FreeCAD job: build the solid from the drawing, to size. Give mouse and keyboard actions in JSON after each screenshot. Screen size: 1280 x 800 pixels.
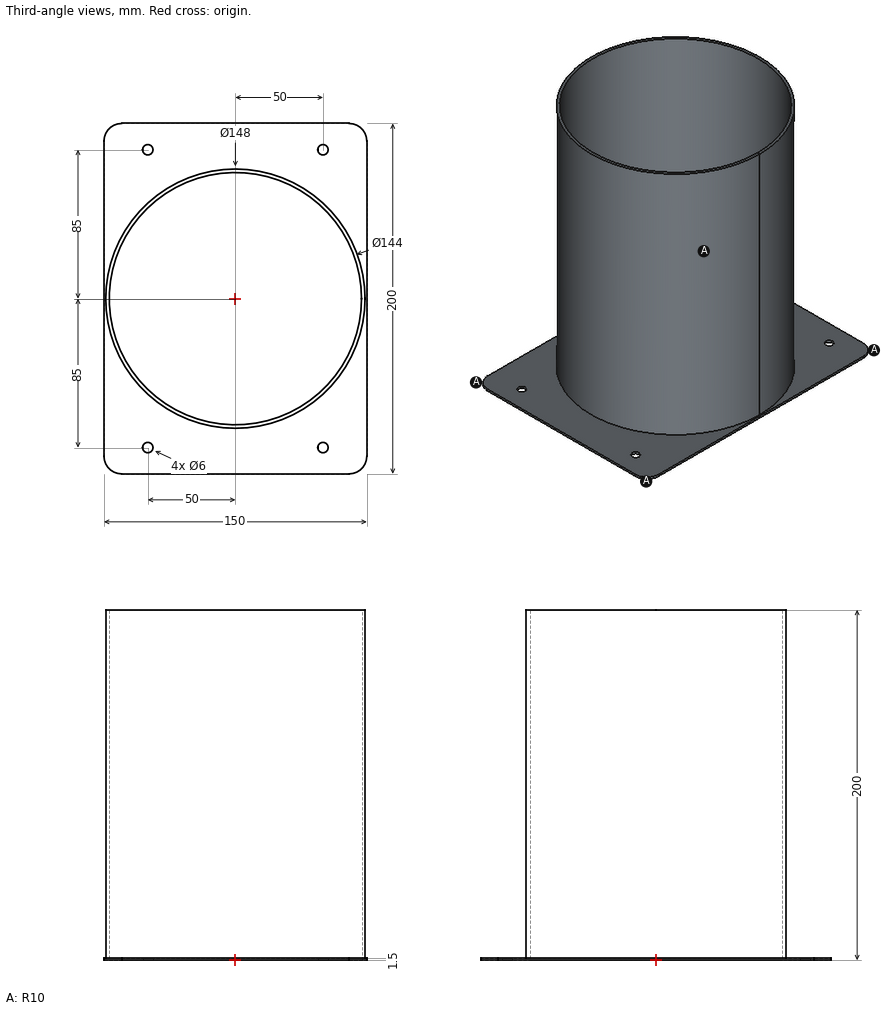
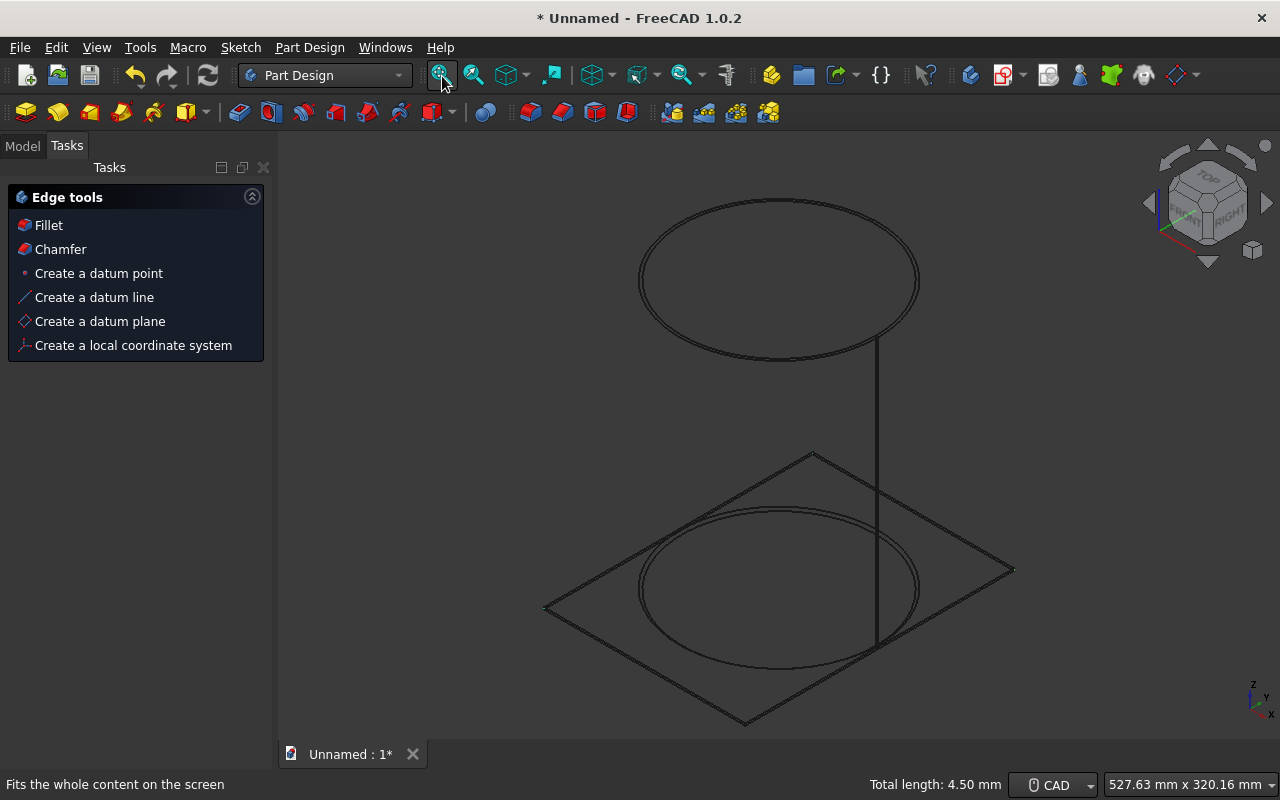
{"action": "key", "text": "2"}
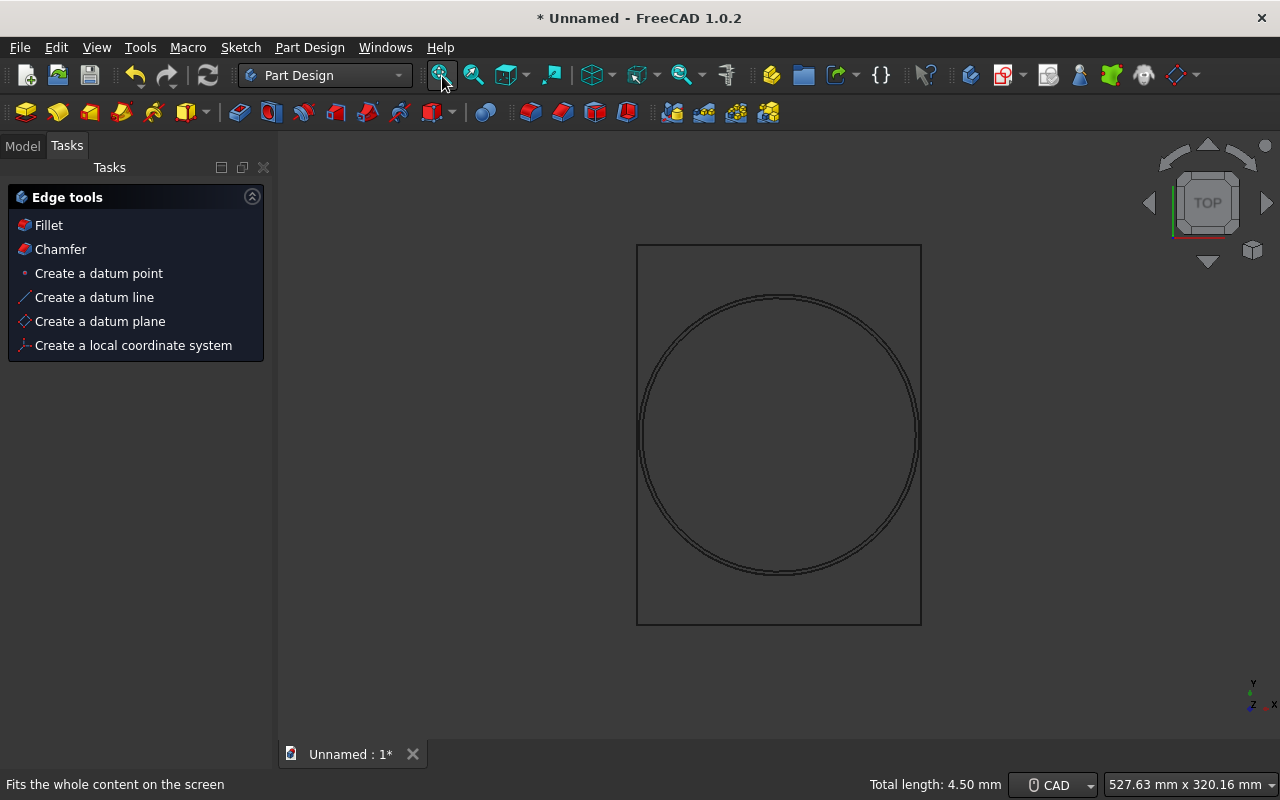
{"action": "scroll", "coordinate": [921, 624], "scroll_direction": "up", "scroll_amount": 14}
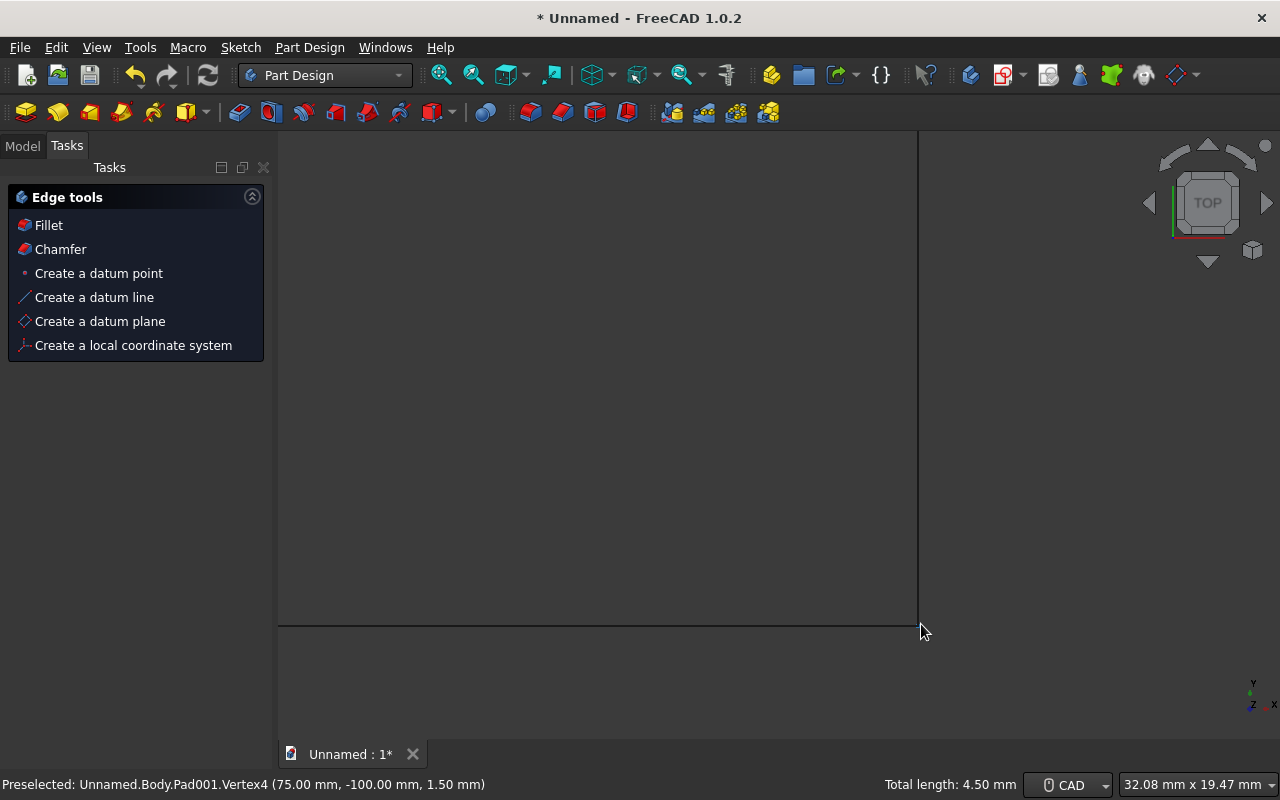
{"action": "left_click", "coordinate": [442, 76]}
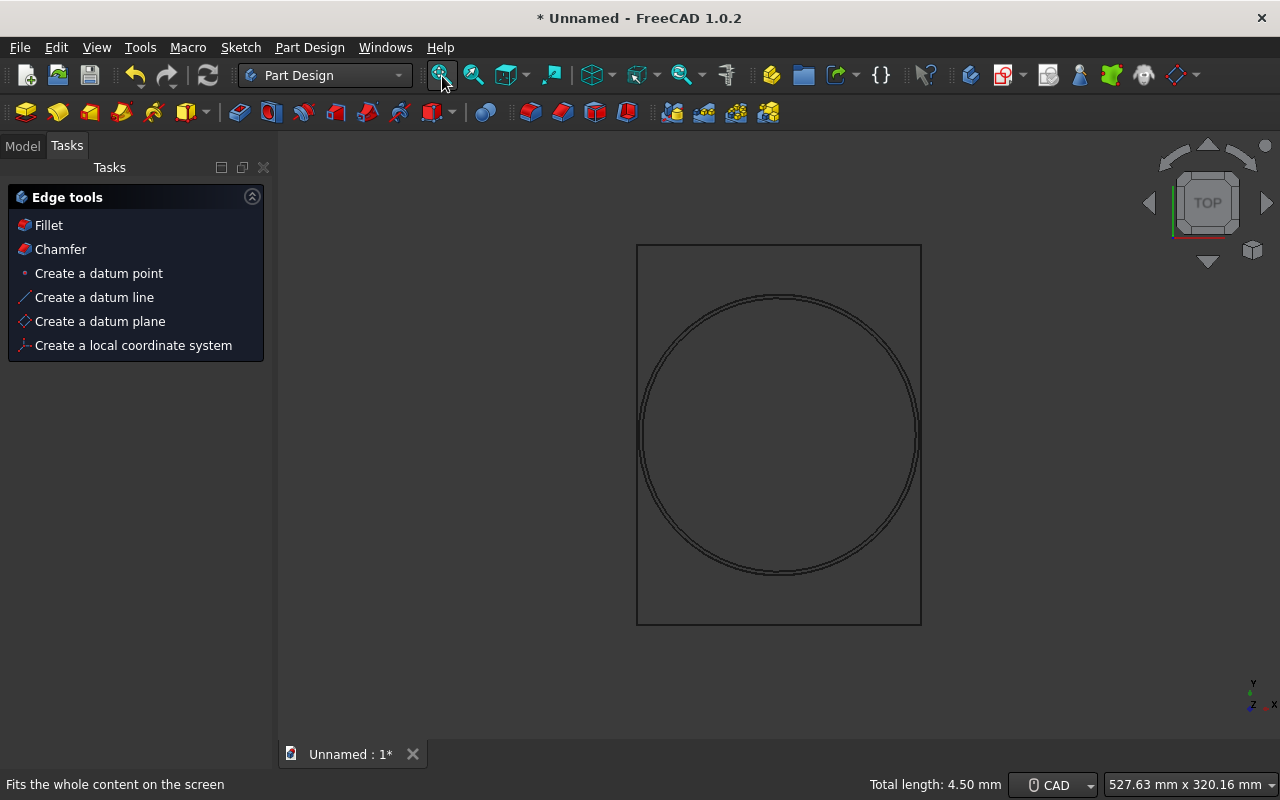
{"action": "key", "text": "1"}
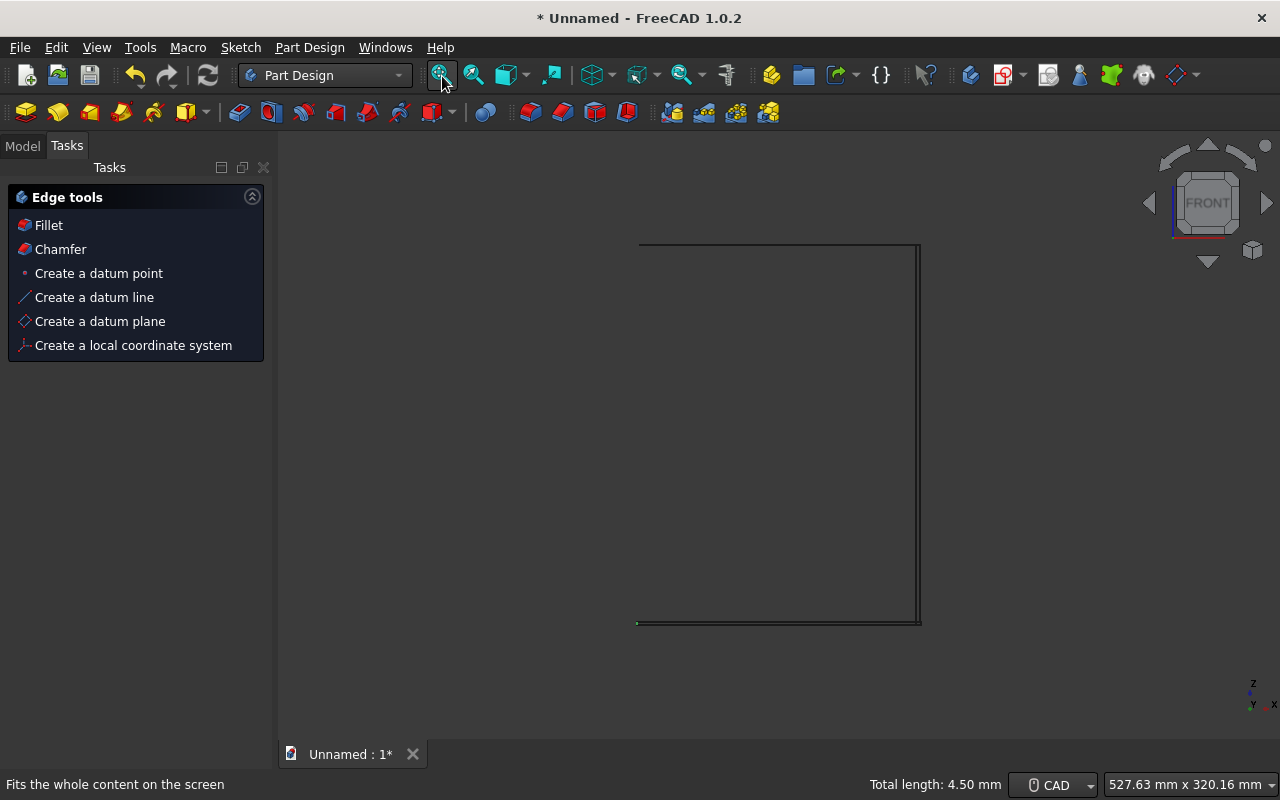
{"action": "scroll", "coordinate": [921, 622], "scroll_direction": "up", "scroll_amount": 14}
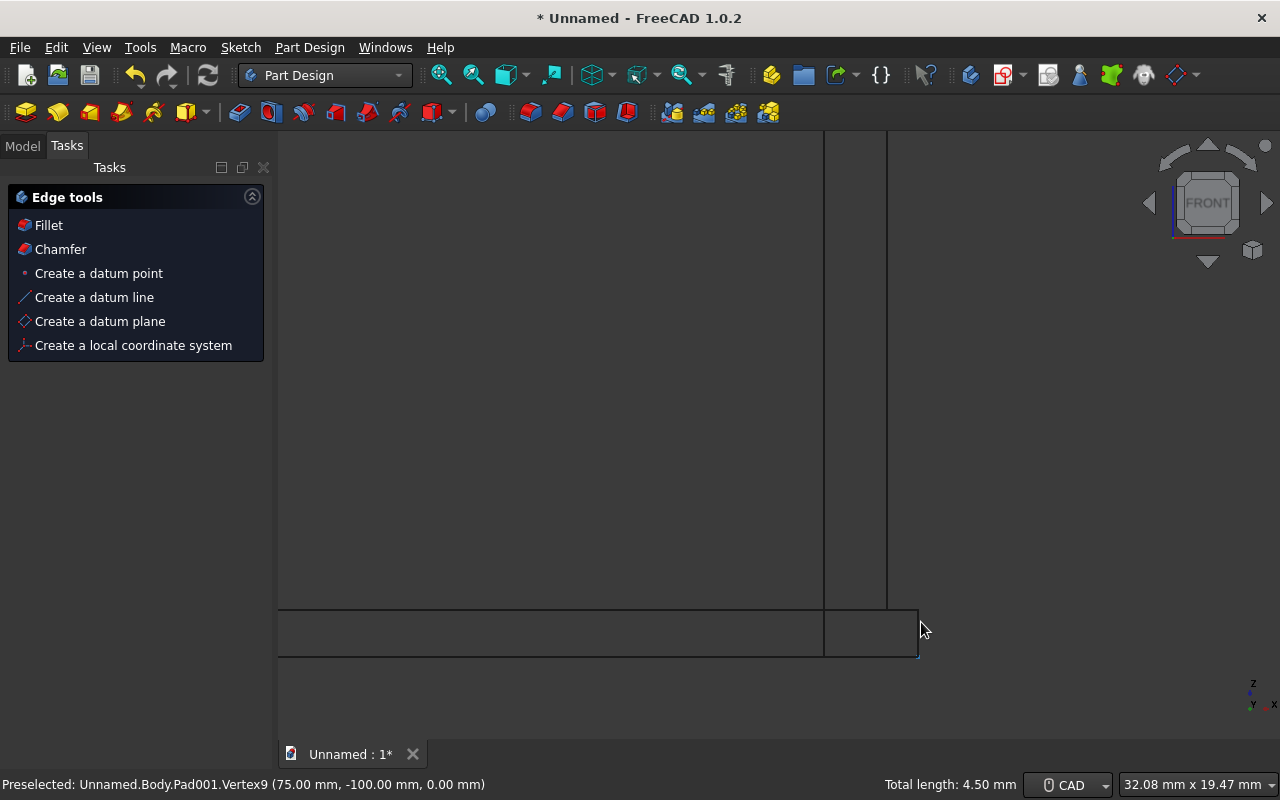
{"action": "left_click", "coordinate": [918, 633], "text": "ctrl"}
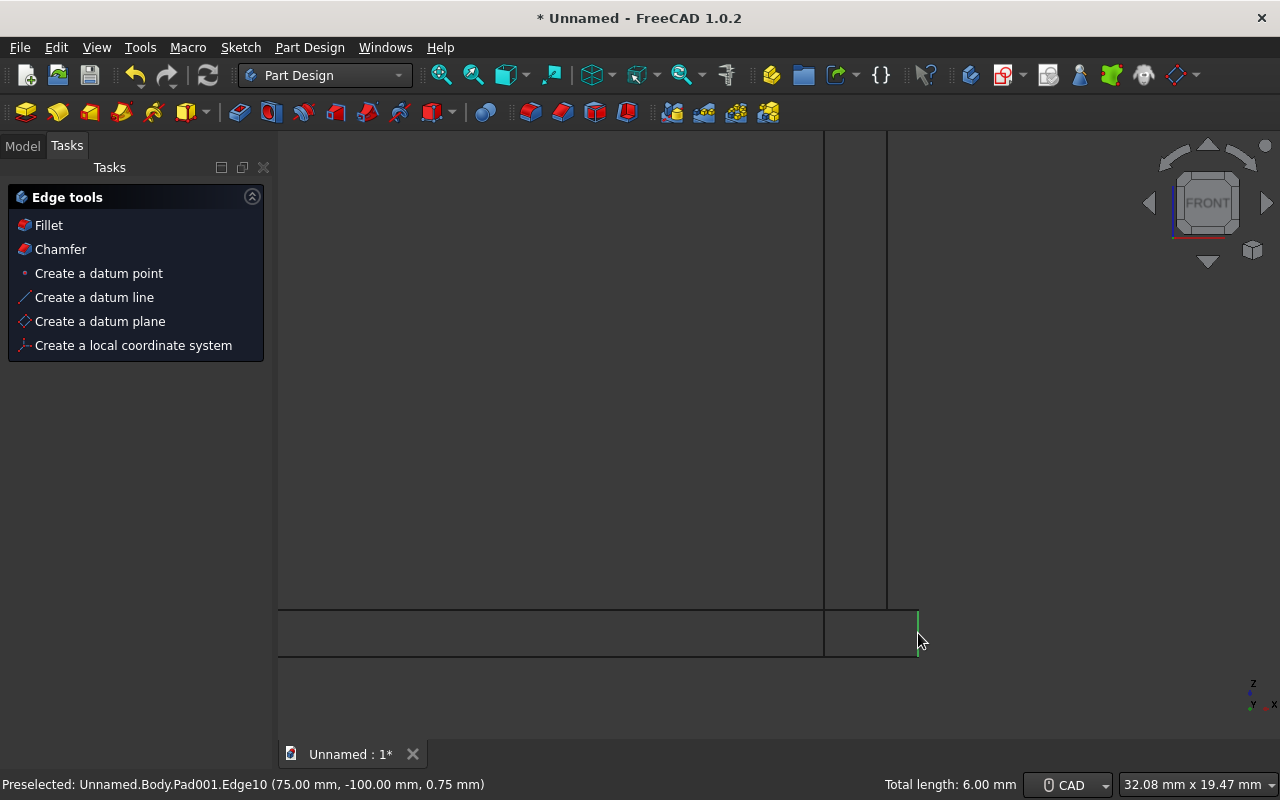
{"action": "key", "text": "v 1"}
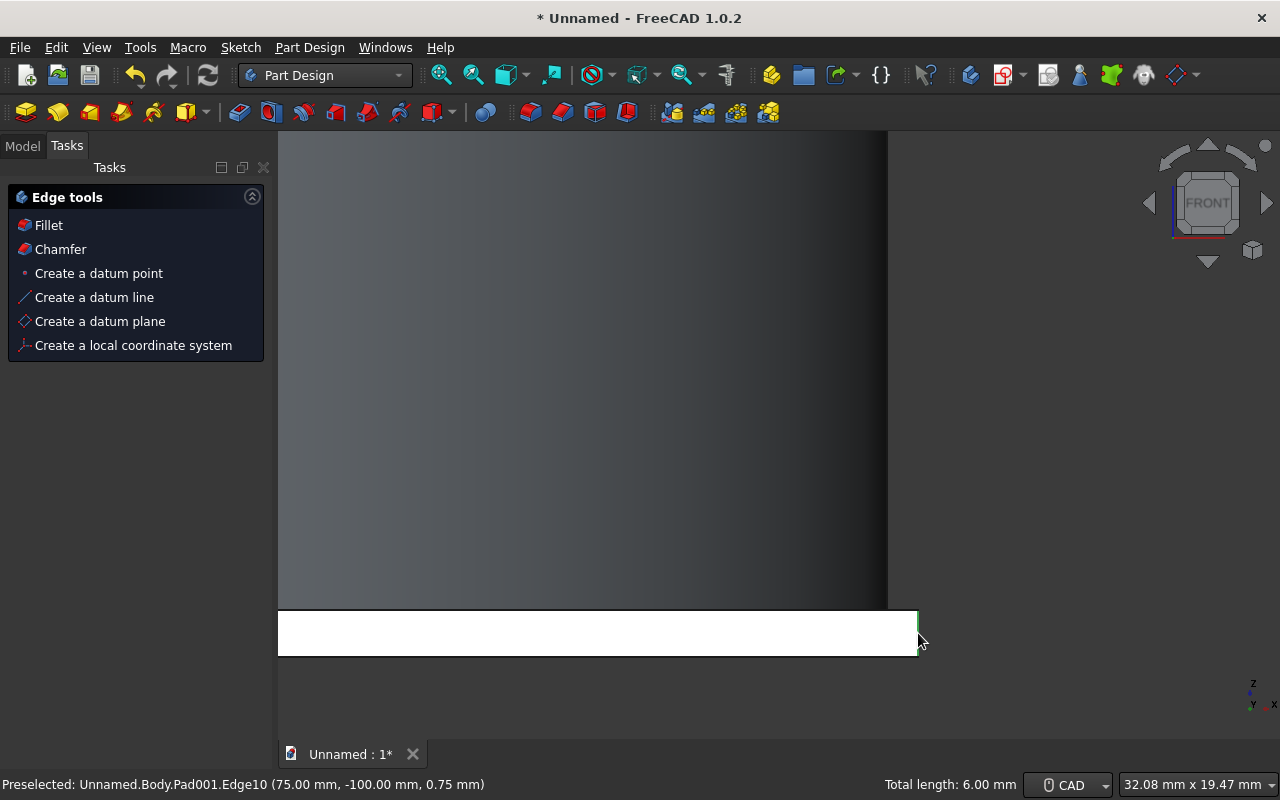
{"action": "left_click", "coordinate": [532, 112]}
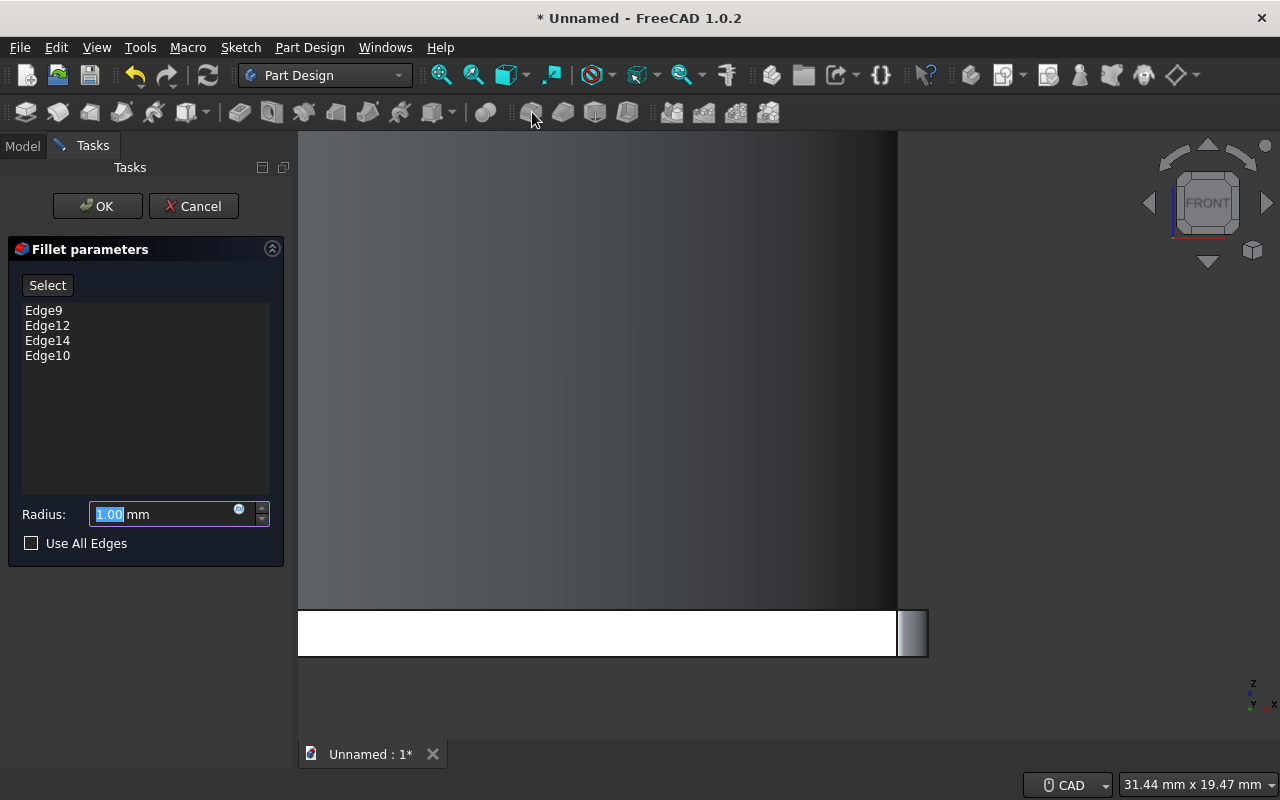
{"action": "type", "text": "10"}
{"action": "key", "text": "Tab"}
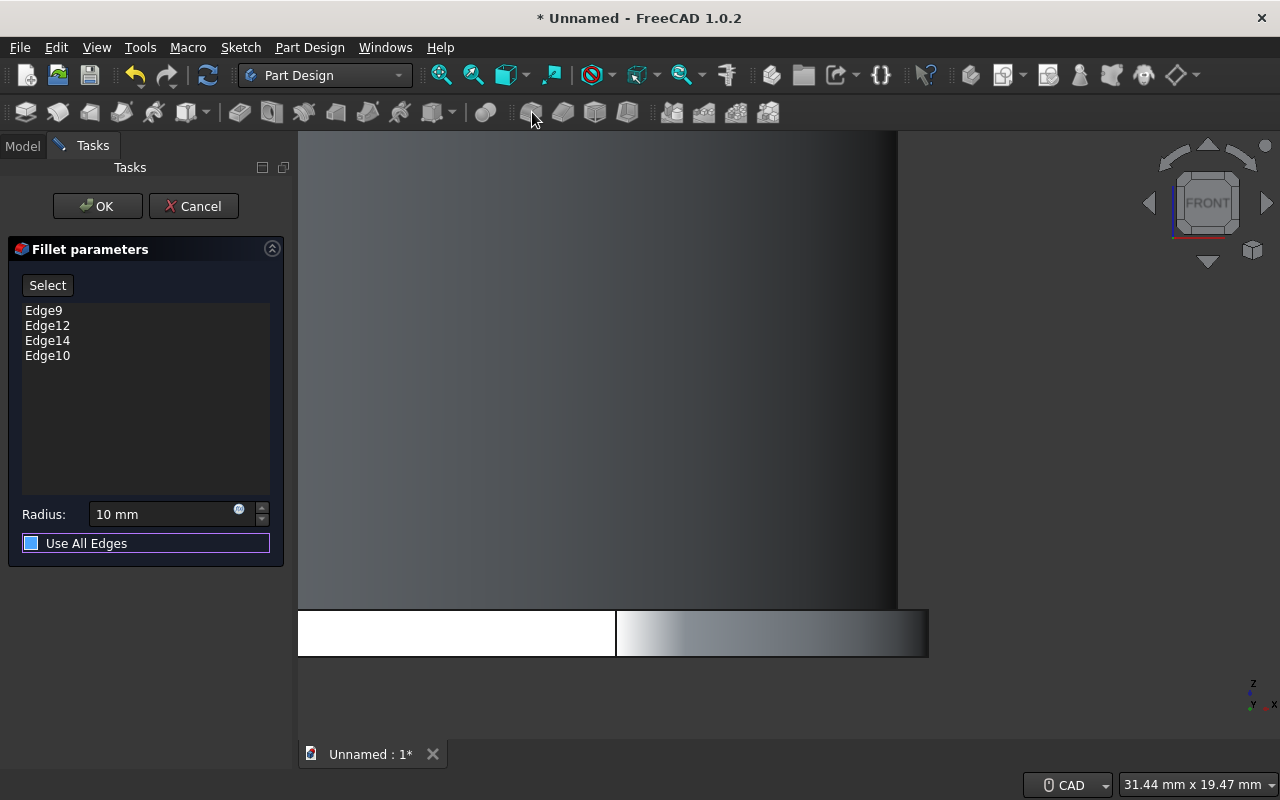
{"action": "left_click", "coordinate": [98, 206]}